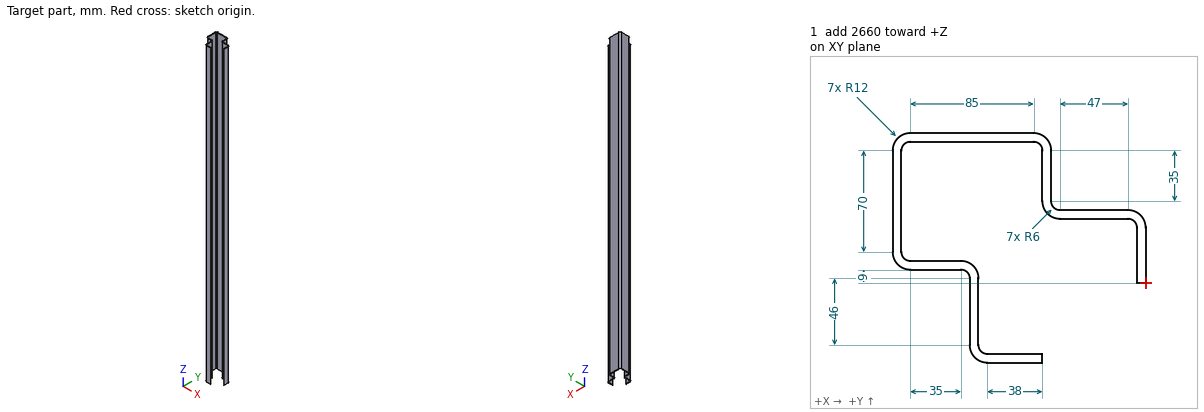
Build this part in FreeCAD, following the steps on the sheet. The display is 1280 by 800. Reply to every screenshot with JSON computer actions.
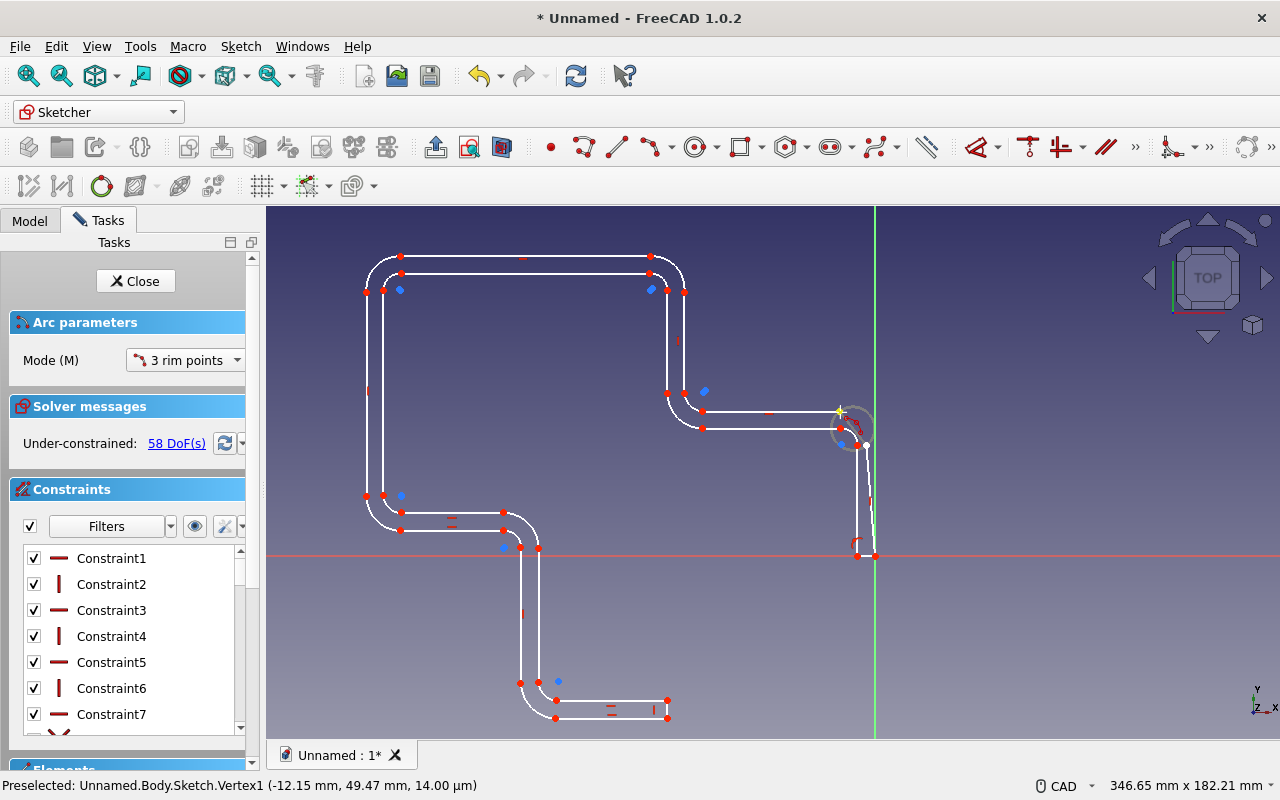
{"action": "scroll", "coordinate": [865, 420], "scroll_direction": "up", "scroll_amount": 3}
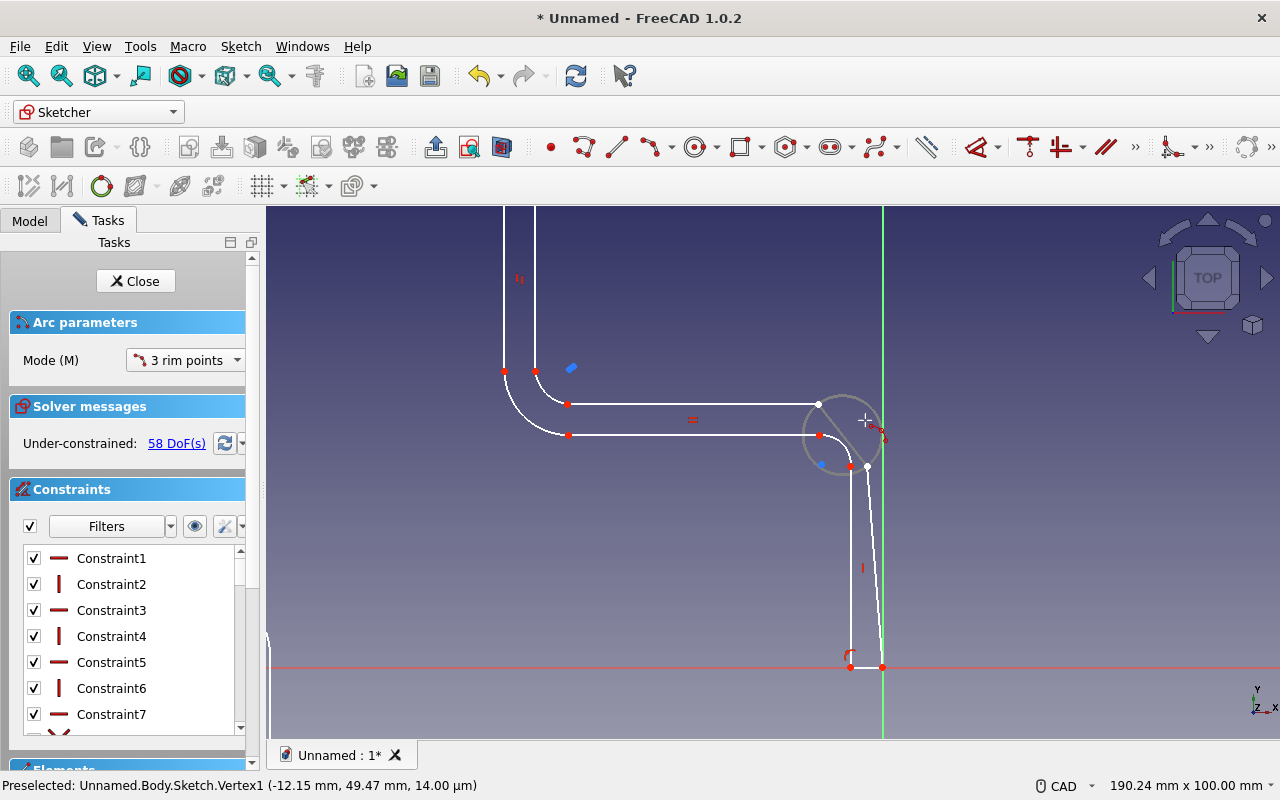
{"action": "left_click", "coordinate": [864, 420]}
{"action": "key", "text": "Escape"}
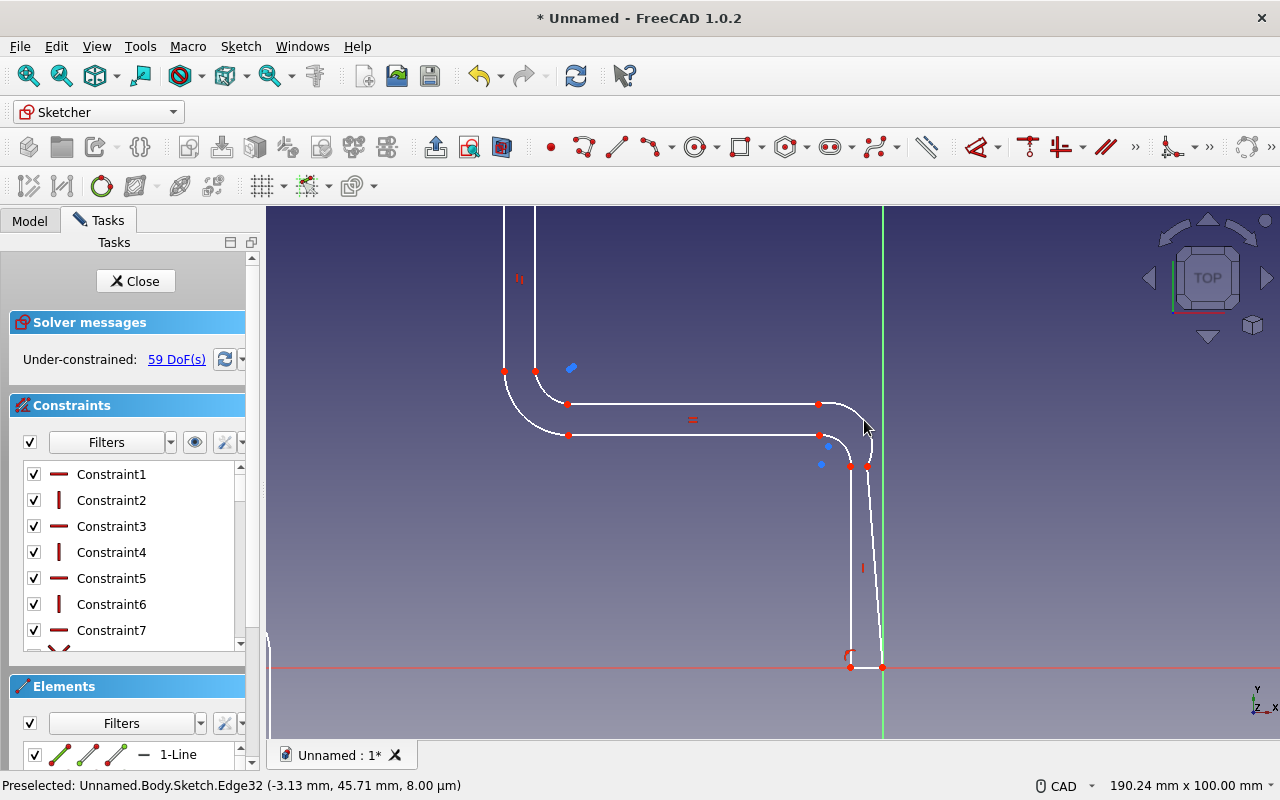
{"action": "left_click", "coordinate": [743, 404]}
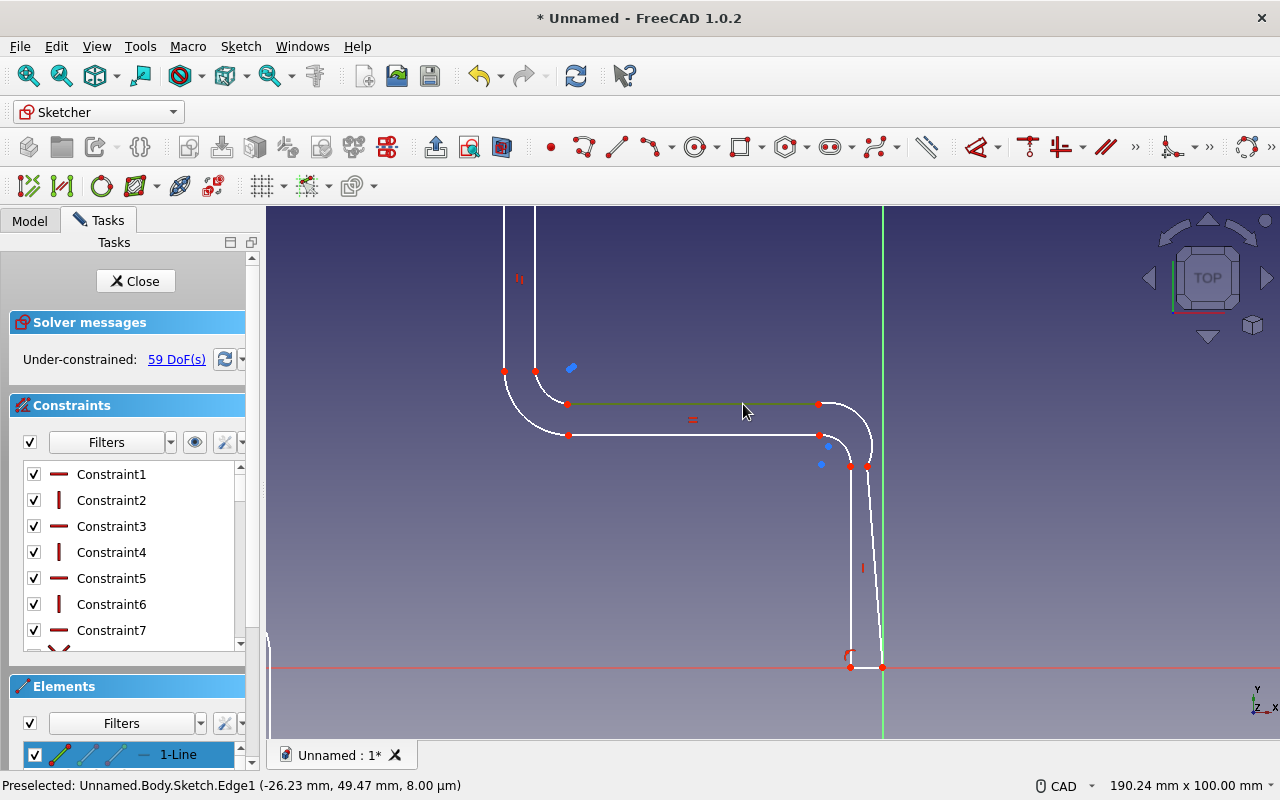
{"action": "left_click", "coordinate": [540, 386]}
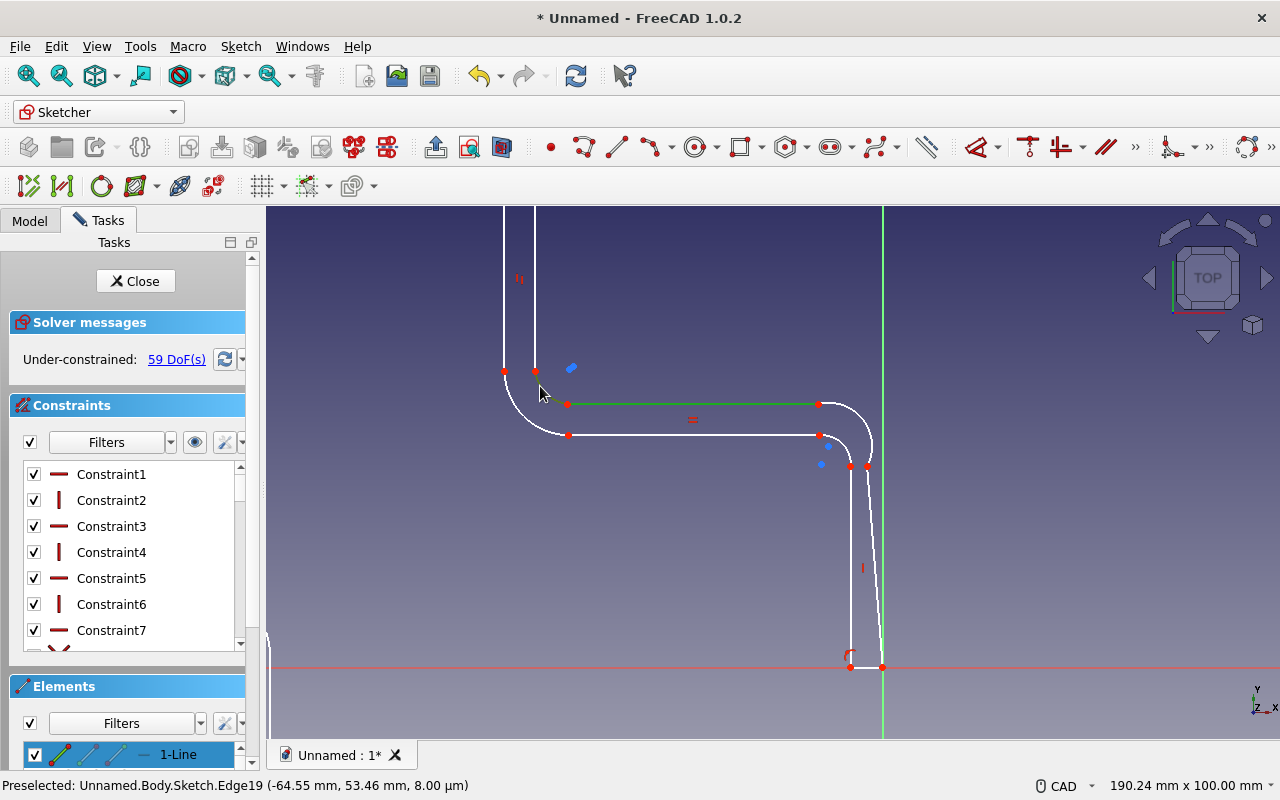
{"action": "key", "text": "t"}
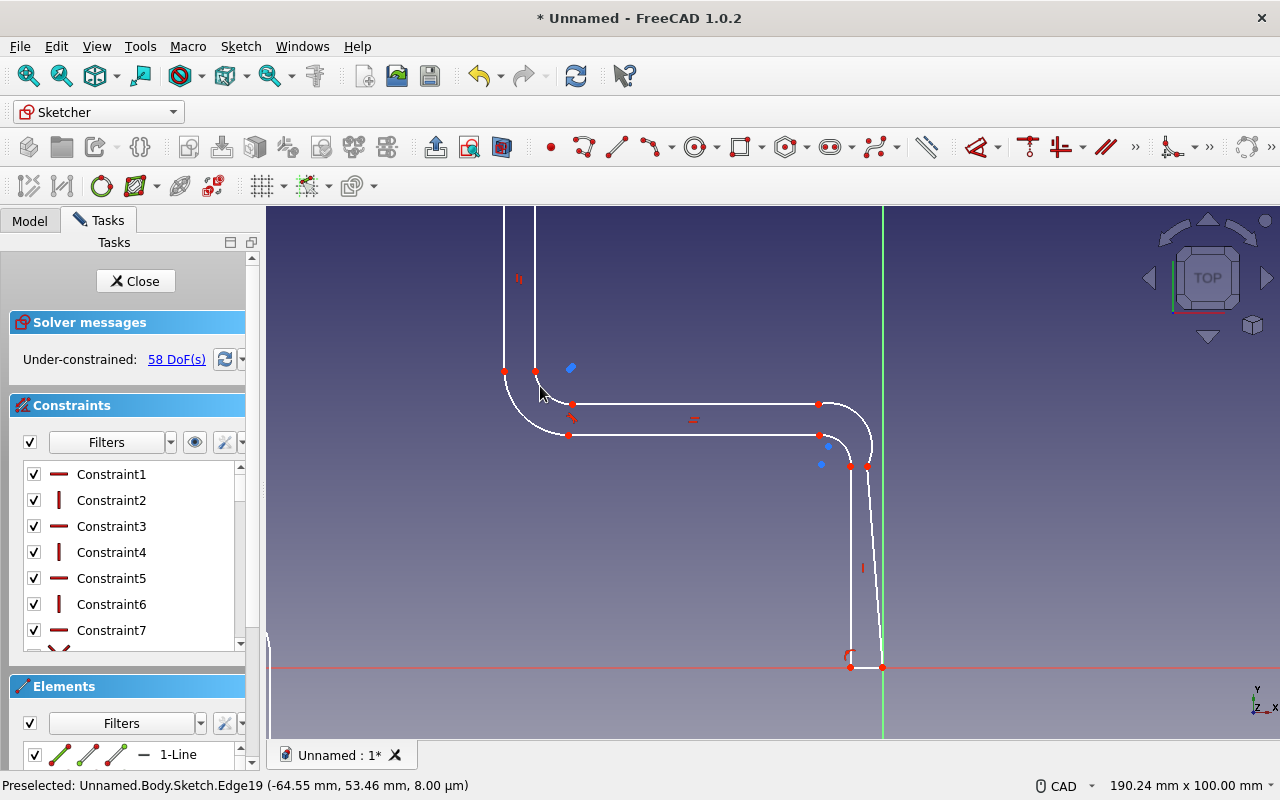
{"action": "left_click", "coordinate": [744, 404]}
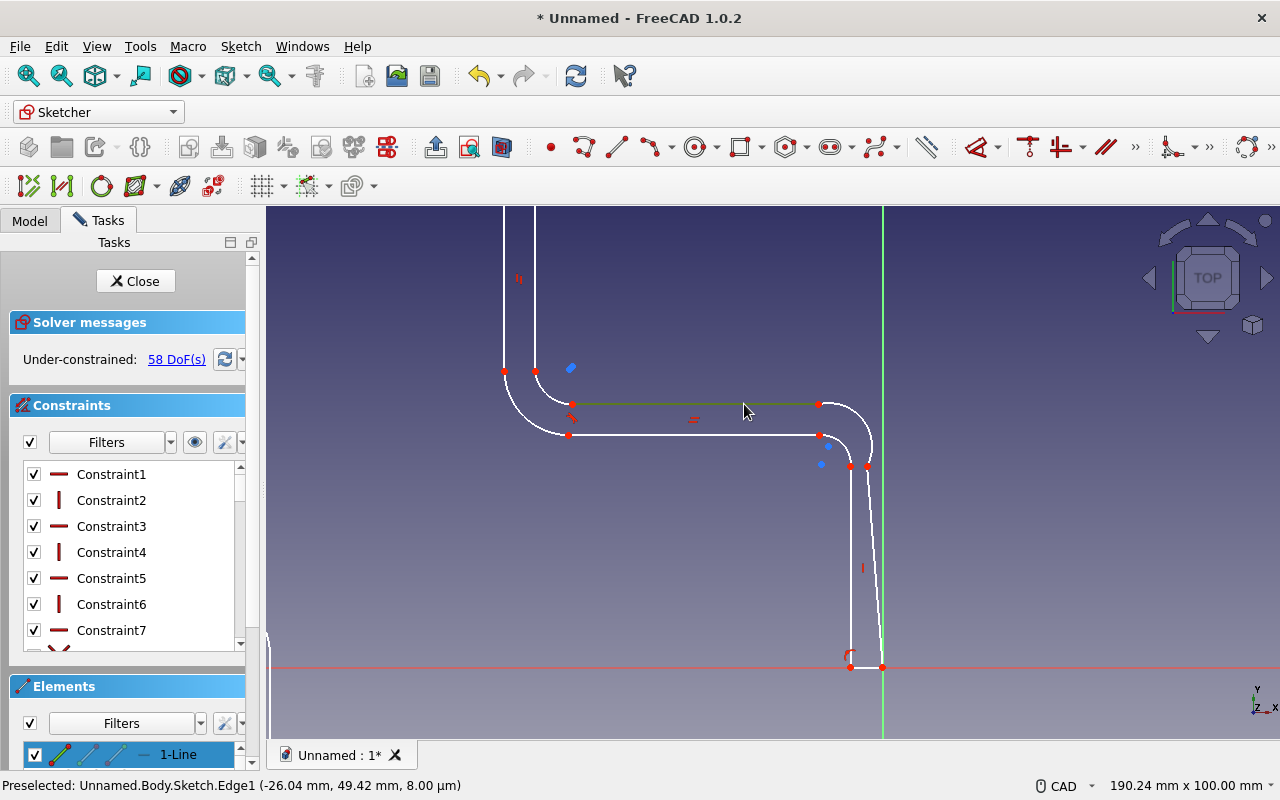
{"action": "left_click", "coordinate": [871, 437]}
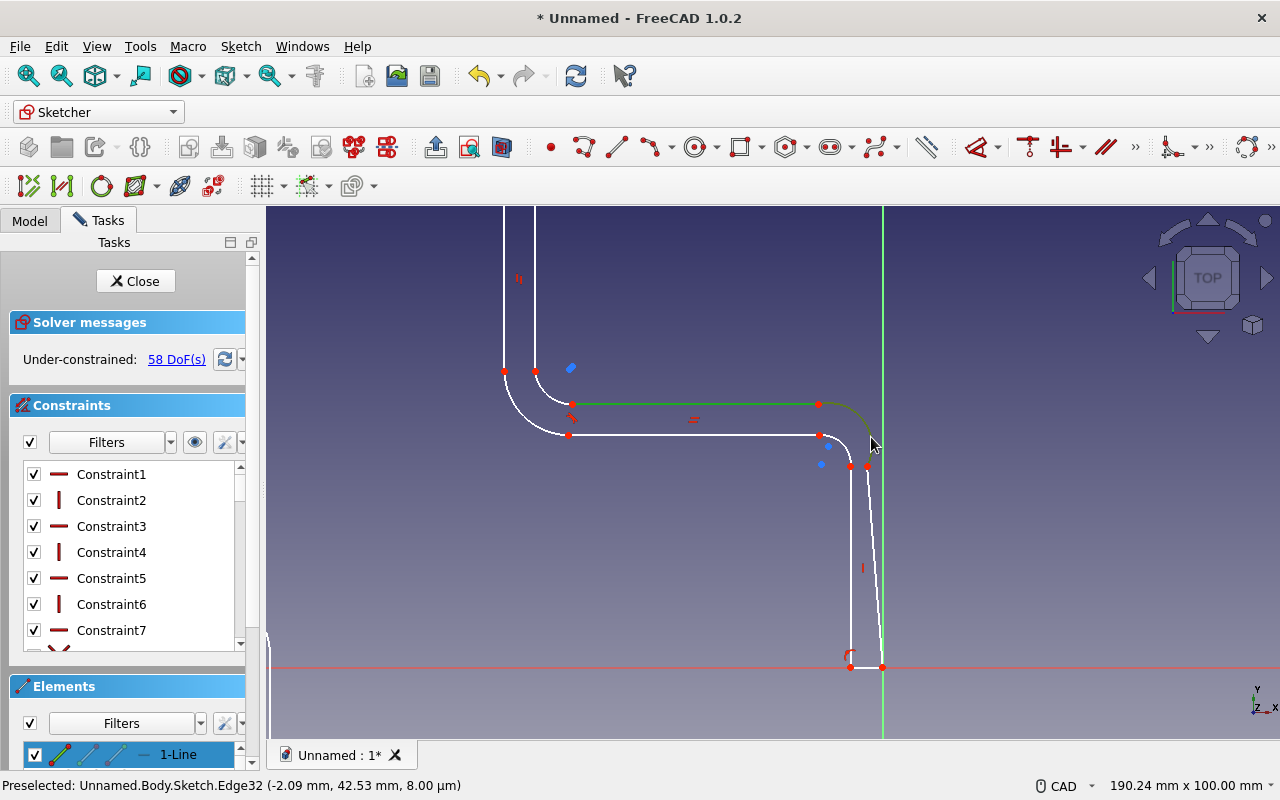
{"action": "key", "text": "t"}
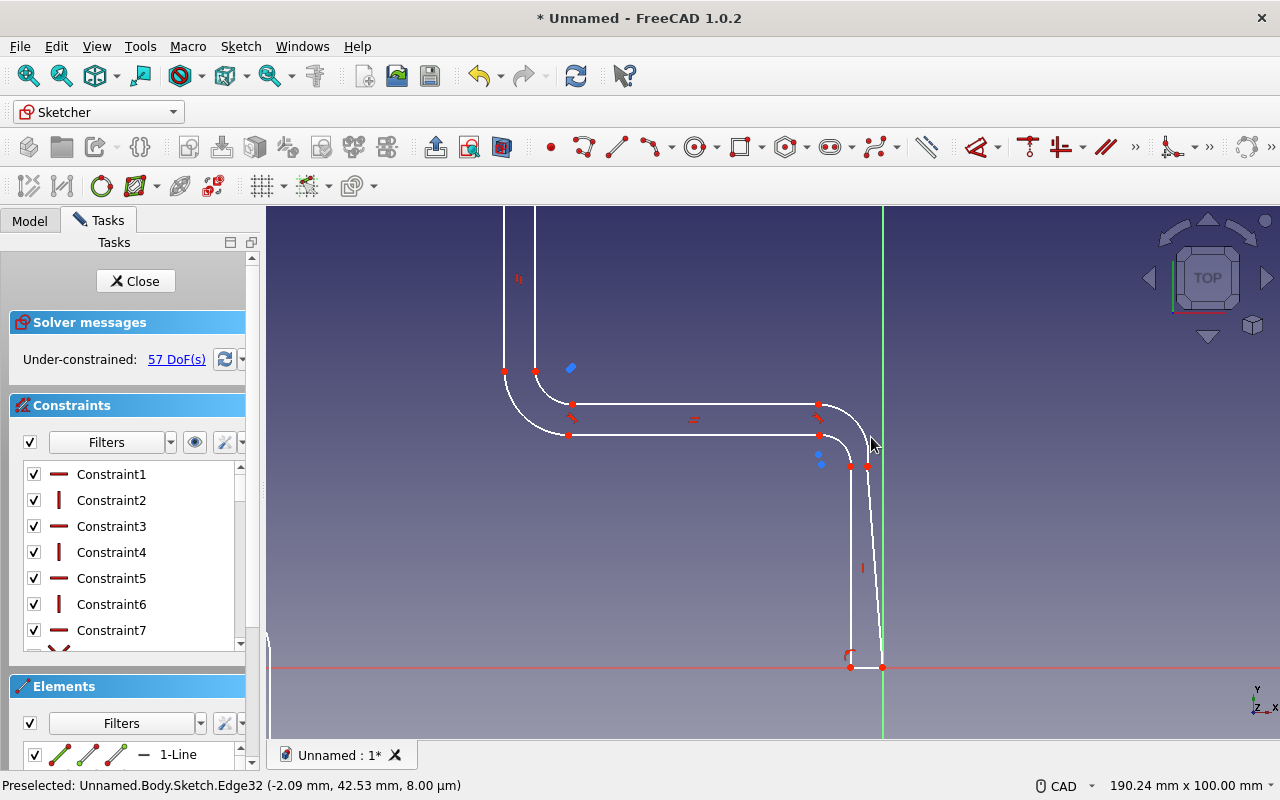
{"action": "left_click", "coordinate": [535, 316]}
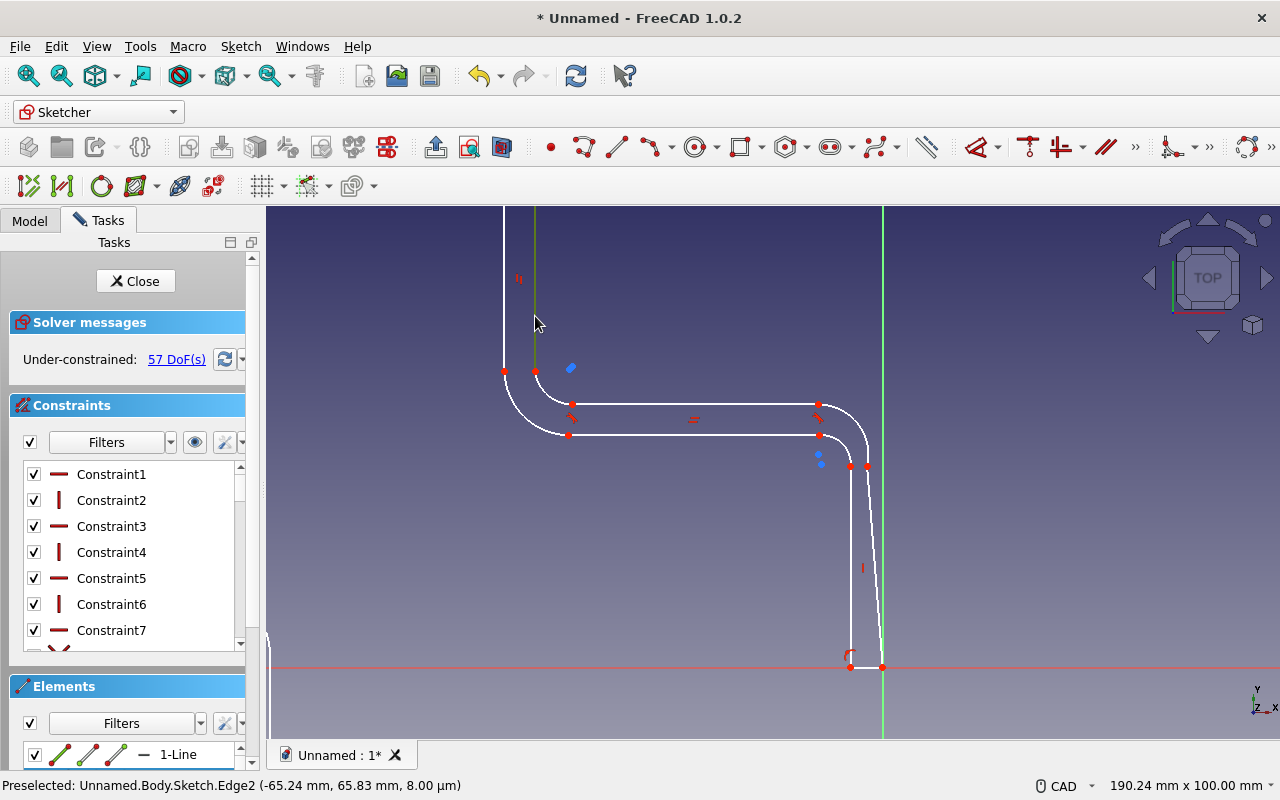
{"action": "left_click", "coordinate": [541, 387]}